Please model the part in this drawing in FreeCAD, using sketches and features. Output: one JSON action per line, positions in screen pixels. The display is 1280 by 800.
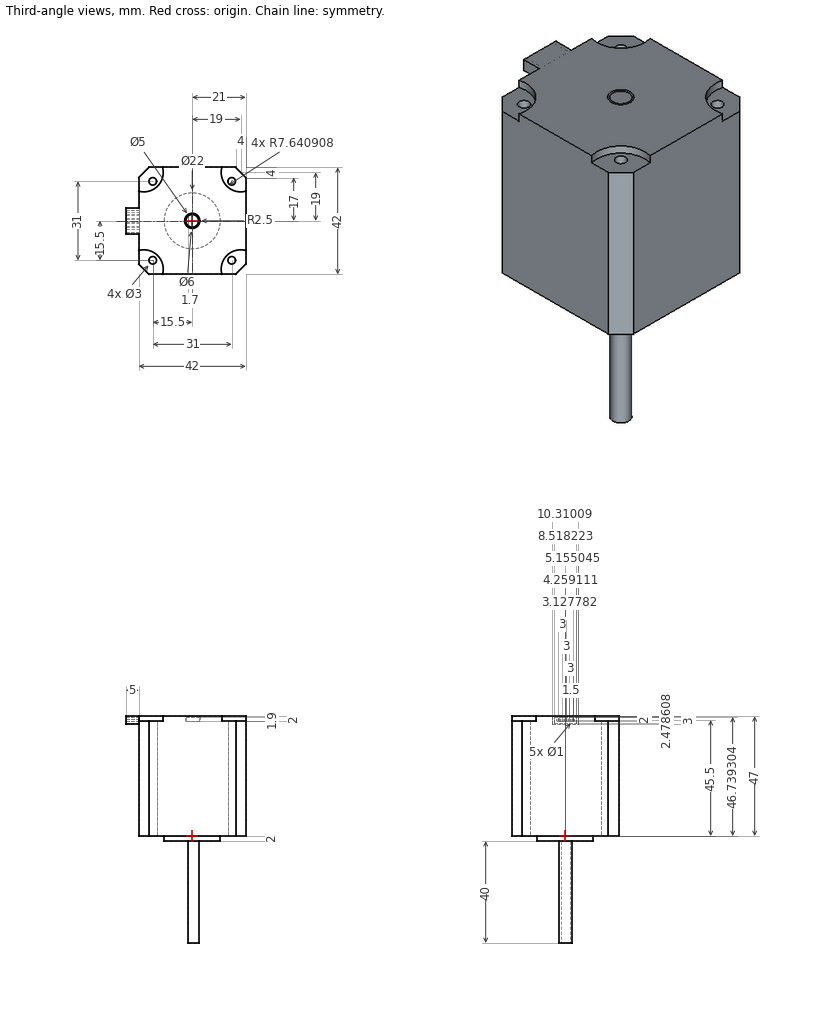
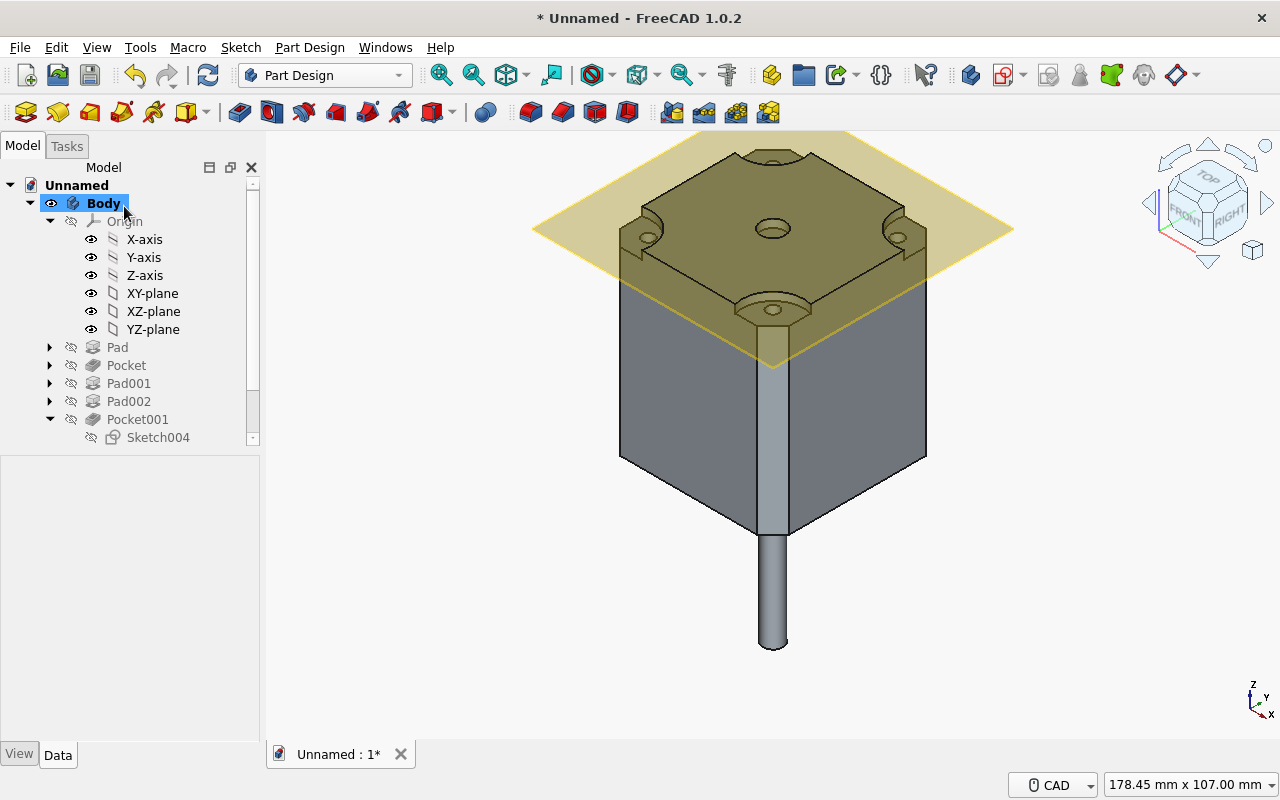
{"action": "scroll", "coordinate": [100, 307], "scroll_direction": "down", "scroll_amount": 3}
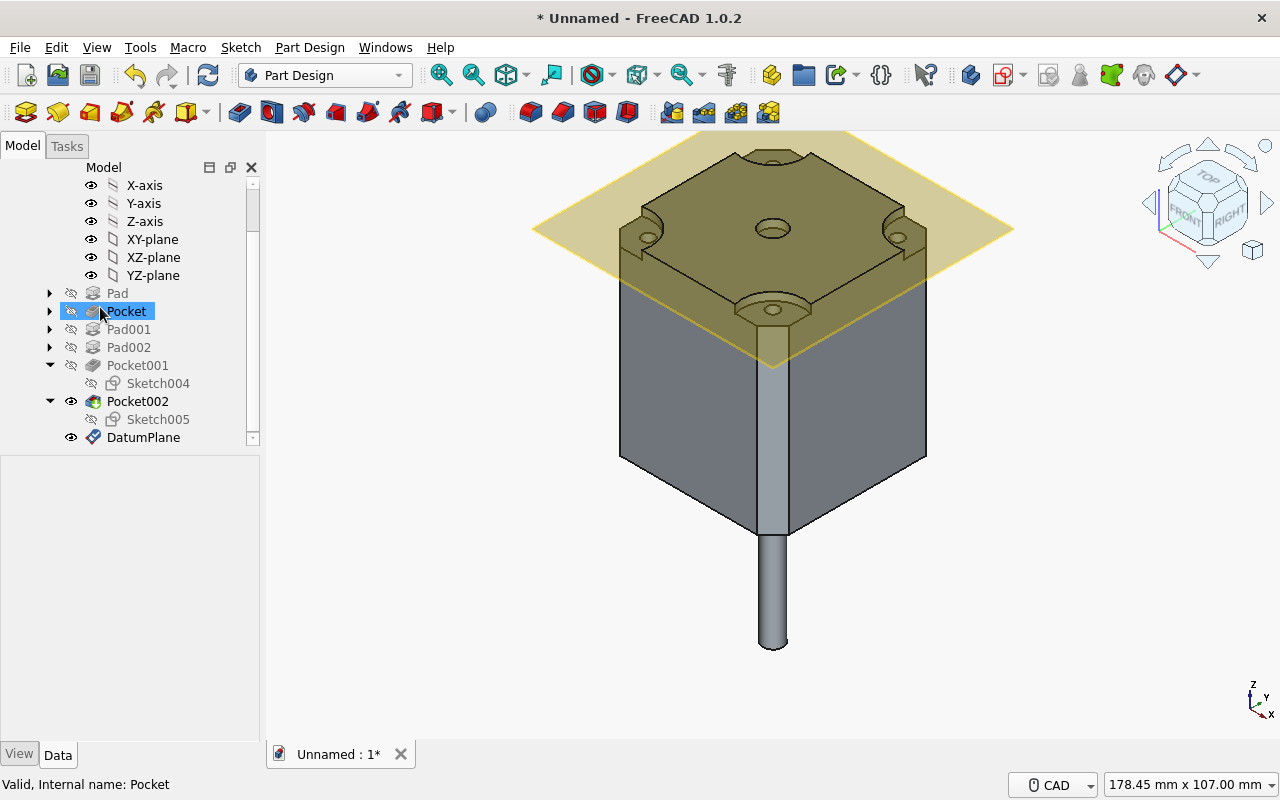
{"action": "left_click", "coordinate": [116, 437]}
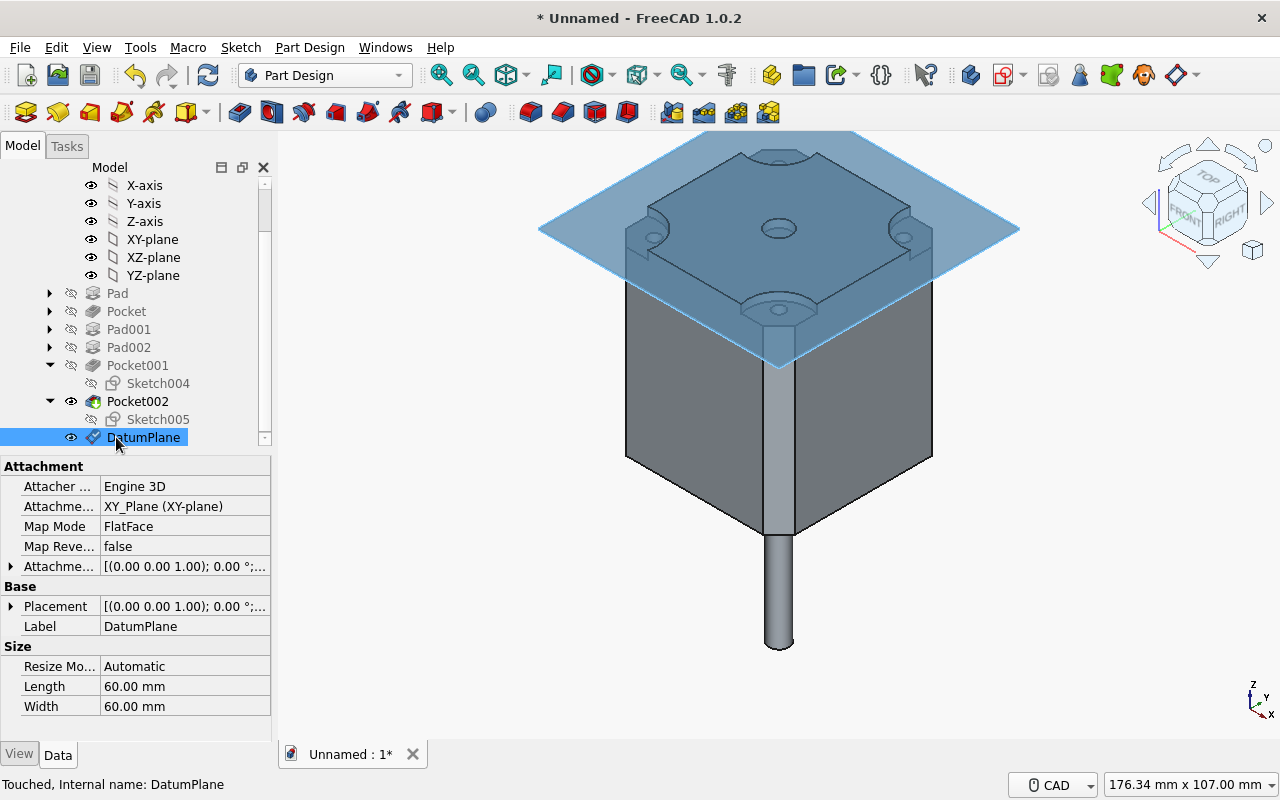
{"action": "left_click", "coordinate": [1004, 76]}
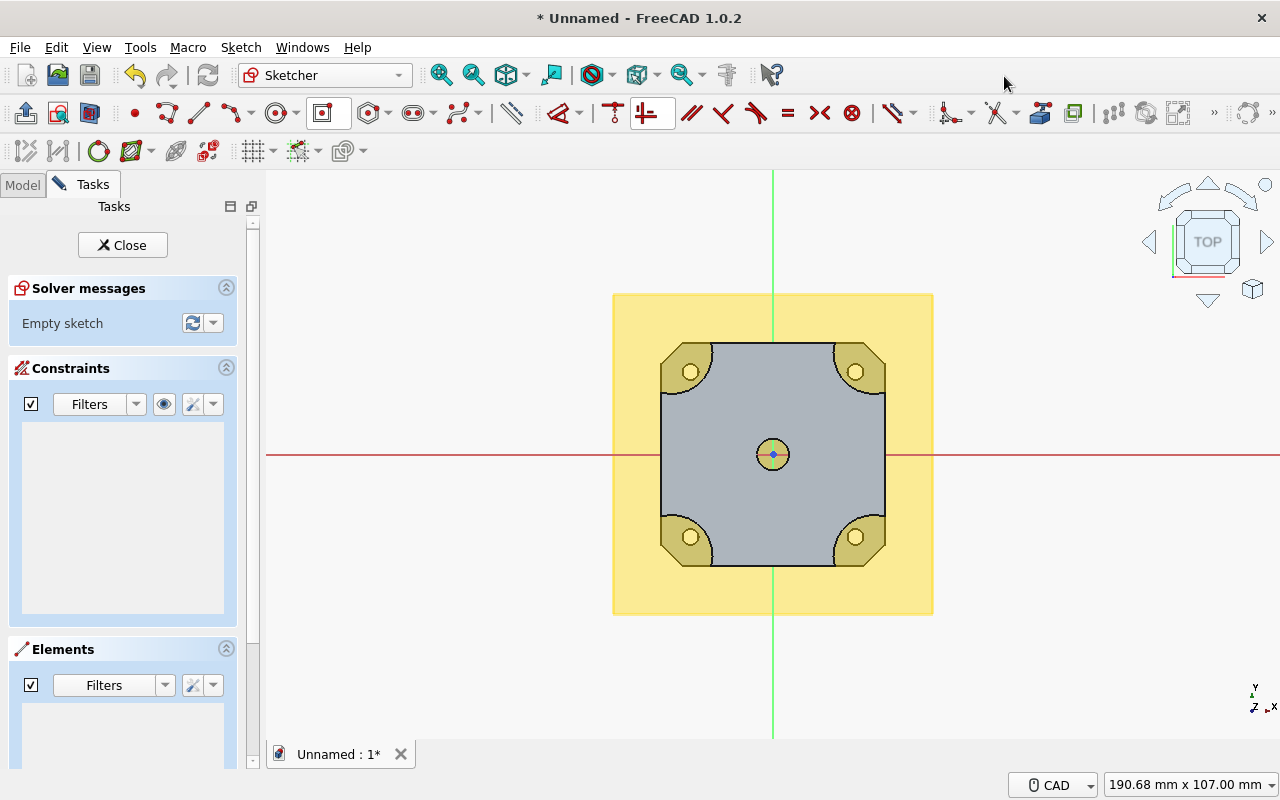
{"action": "left_click", "coordinate": [90, 114]}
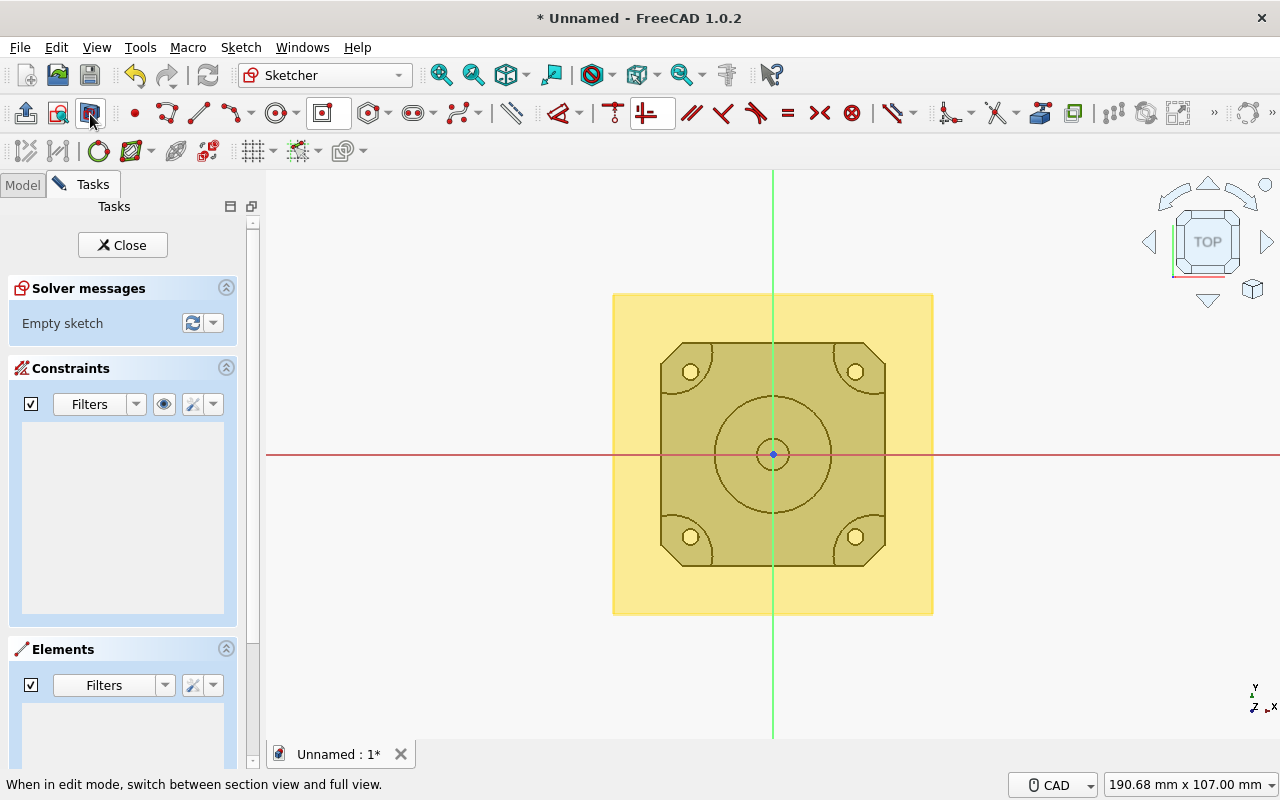
{"action": "scroll", "coordinate": [778, 454], "scroll_direction": "up", "scroll_amount": 13}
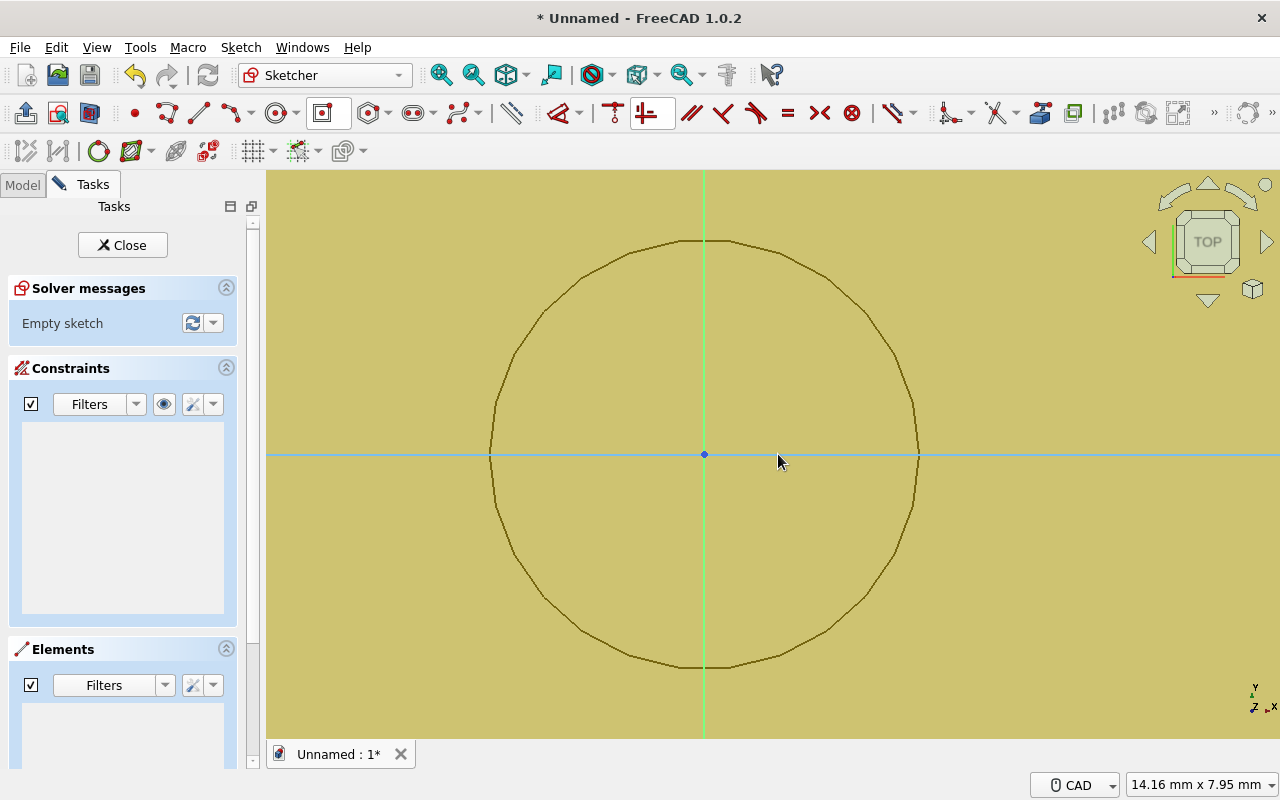
{"action": "left_click", "coordinate": [276, 114]}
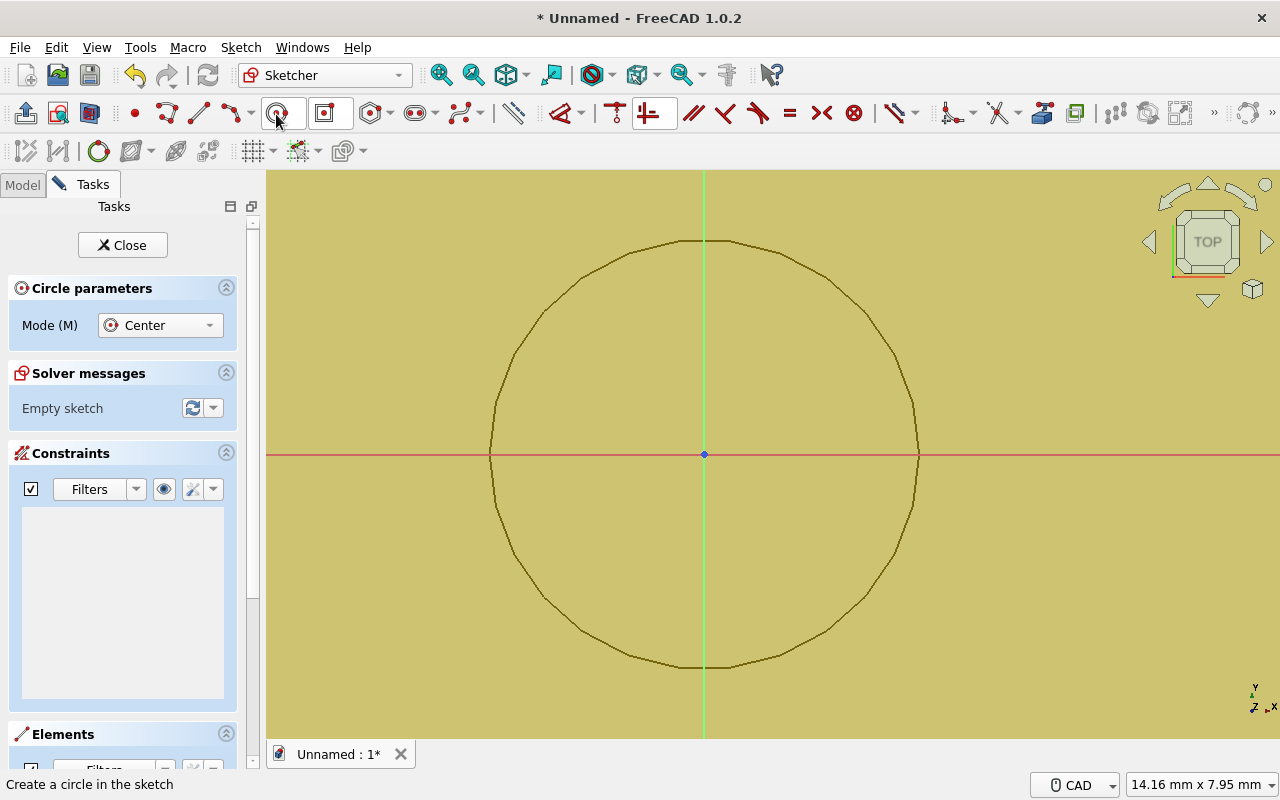
{"action": "left_click", "coordinate": [704, 454]}
{"action": "left_click", "coordinate": [831, 328]}
{"action": "key", "text": "Escape"}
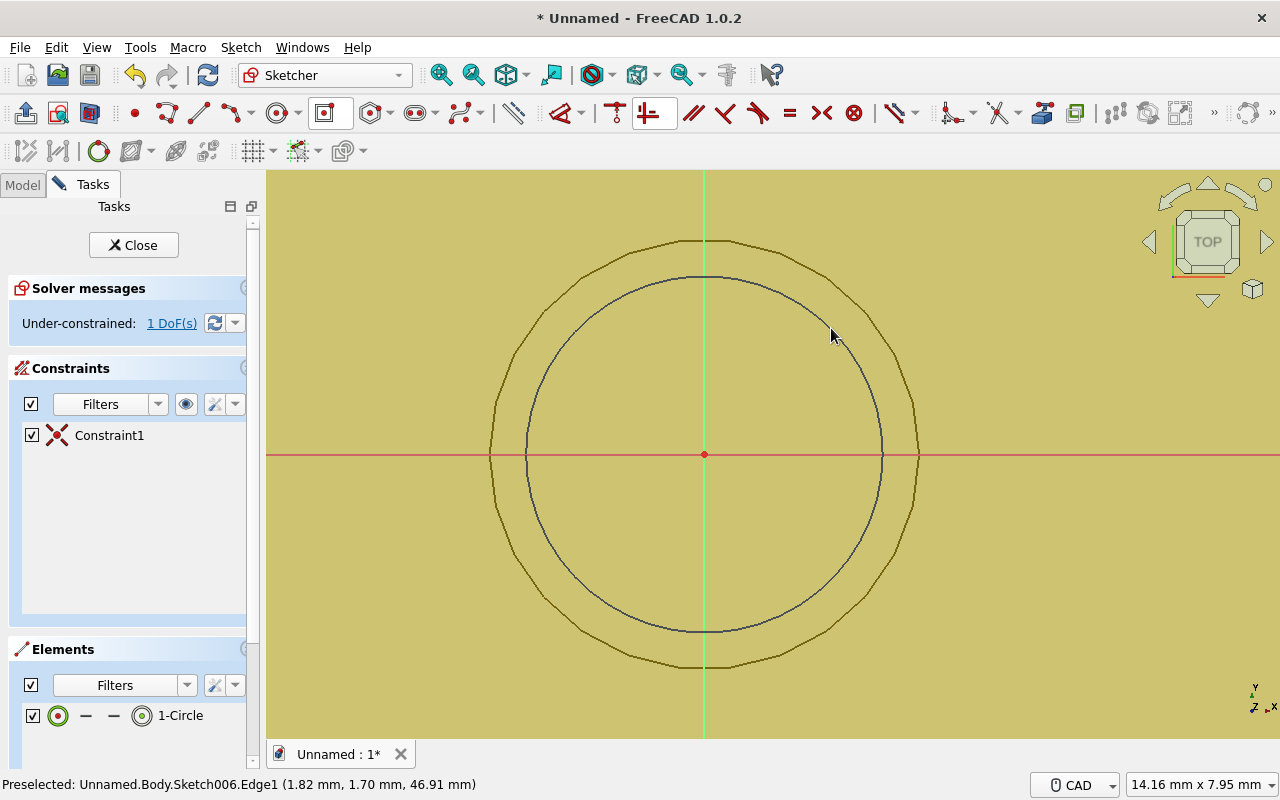
{"action": "left_click", "coordinate": [560, 114]}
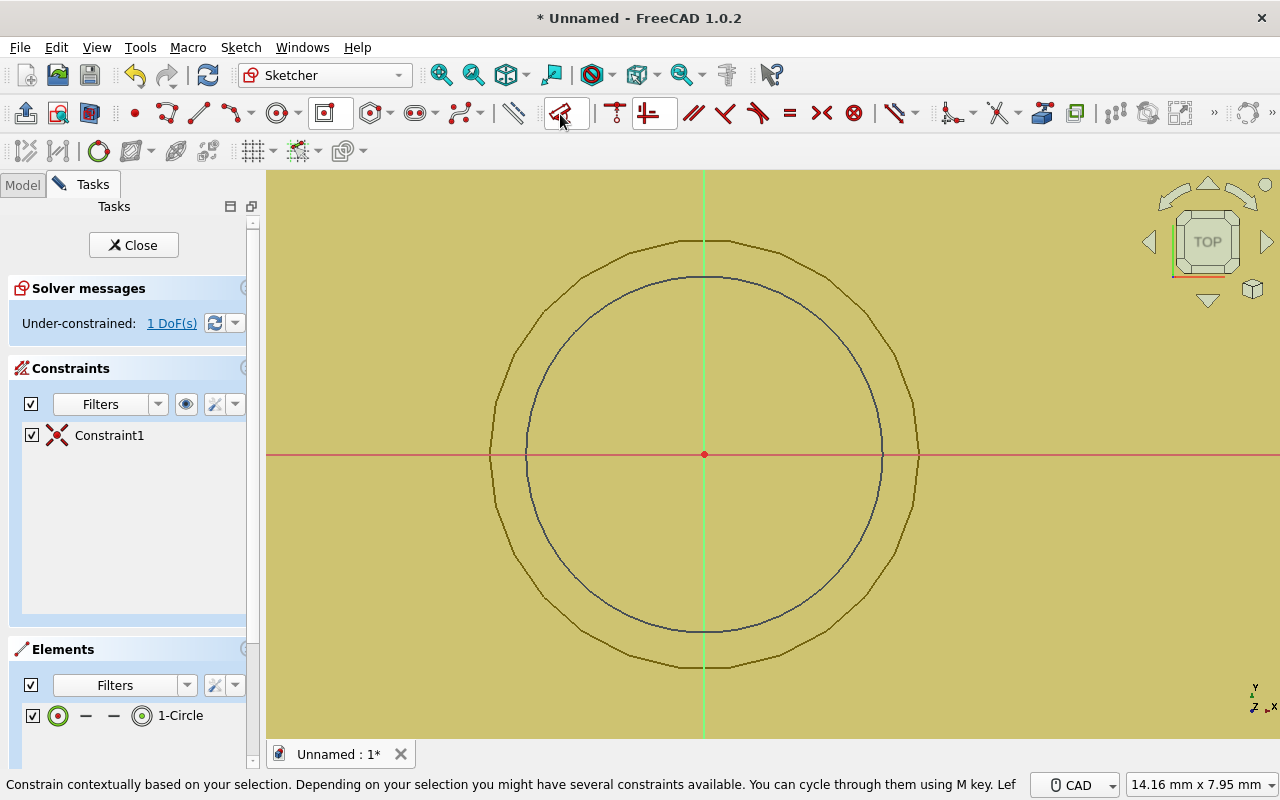
{"action": "left_click", "coordinate": [830, 328]}
{"action": "left_click", "coordinate": [853, 305]}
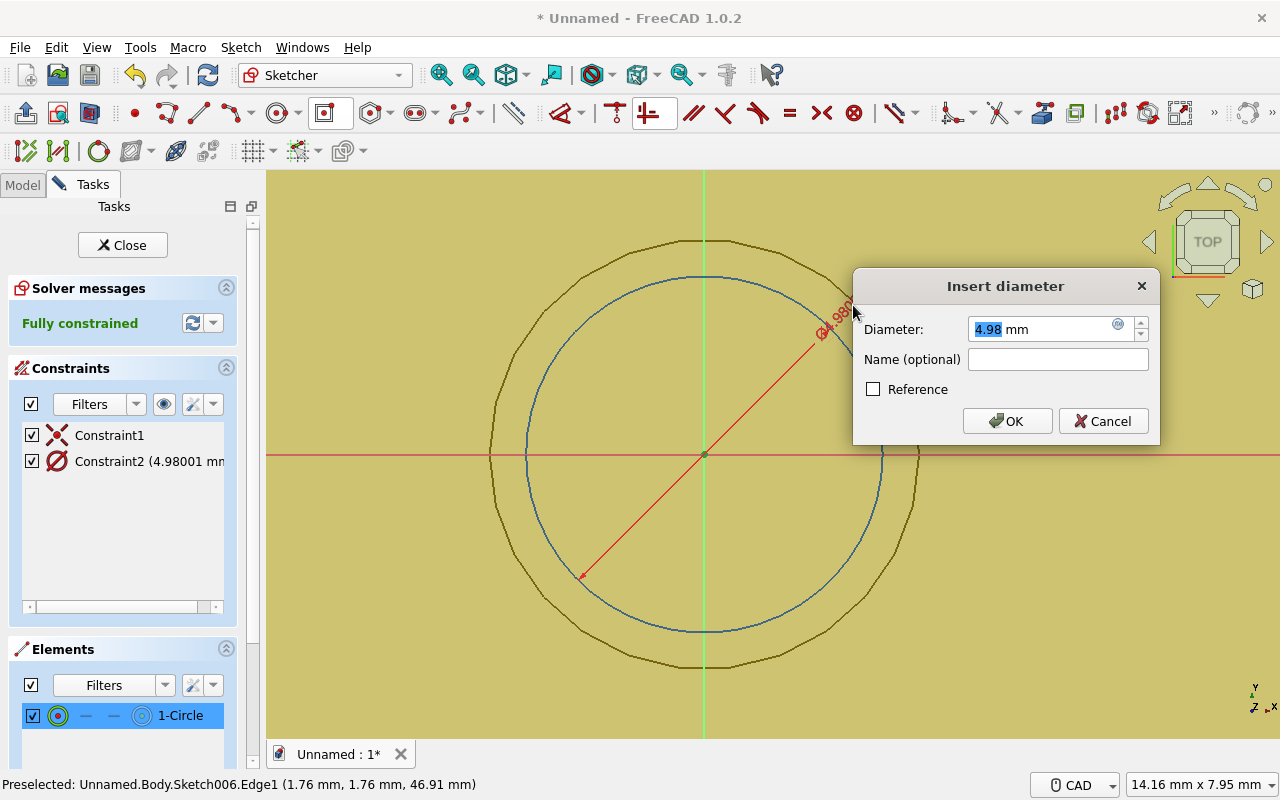
{"action": "type", "text": "5"}
{"action": "key", "text": "Return"}
{"action": "key", "text": "Escape"}